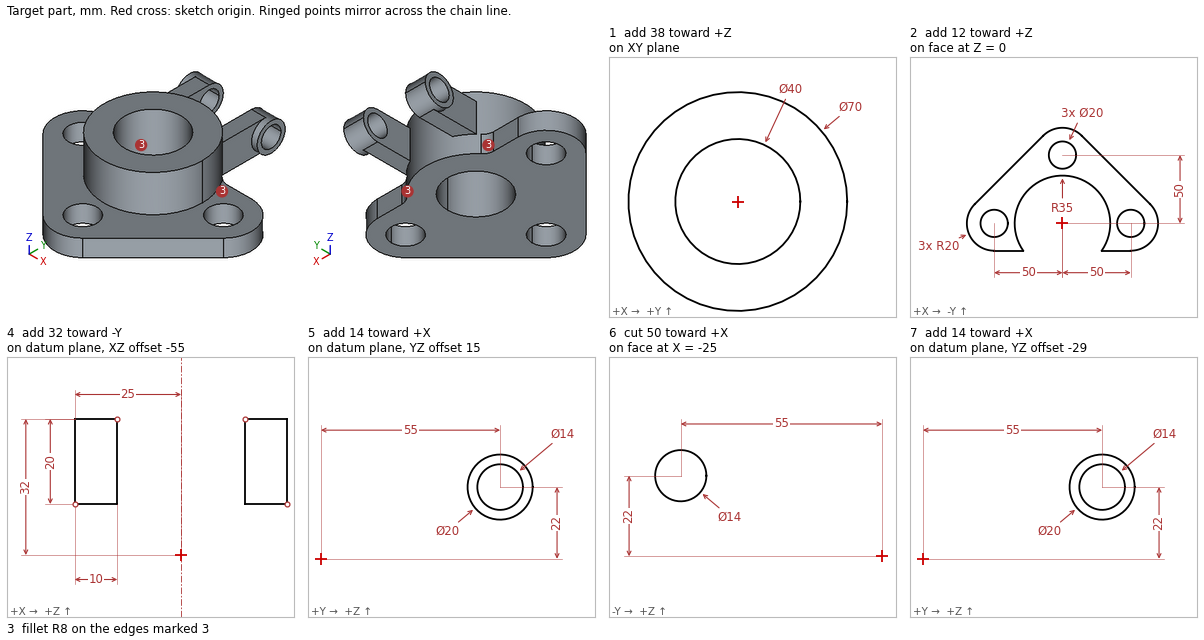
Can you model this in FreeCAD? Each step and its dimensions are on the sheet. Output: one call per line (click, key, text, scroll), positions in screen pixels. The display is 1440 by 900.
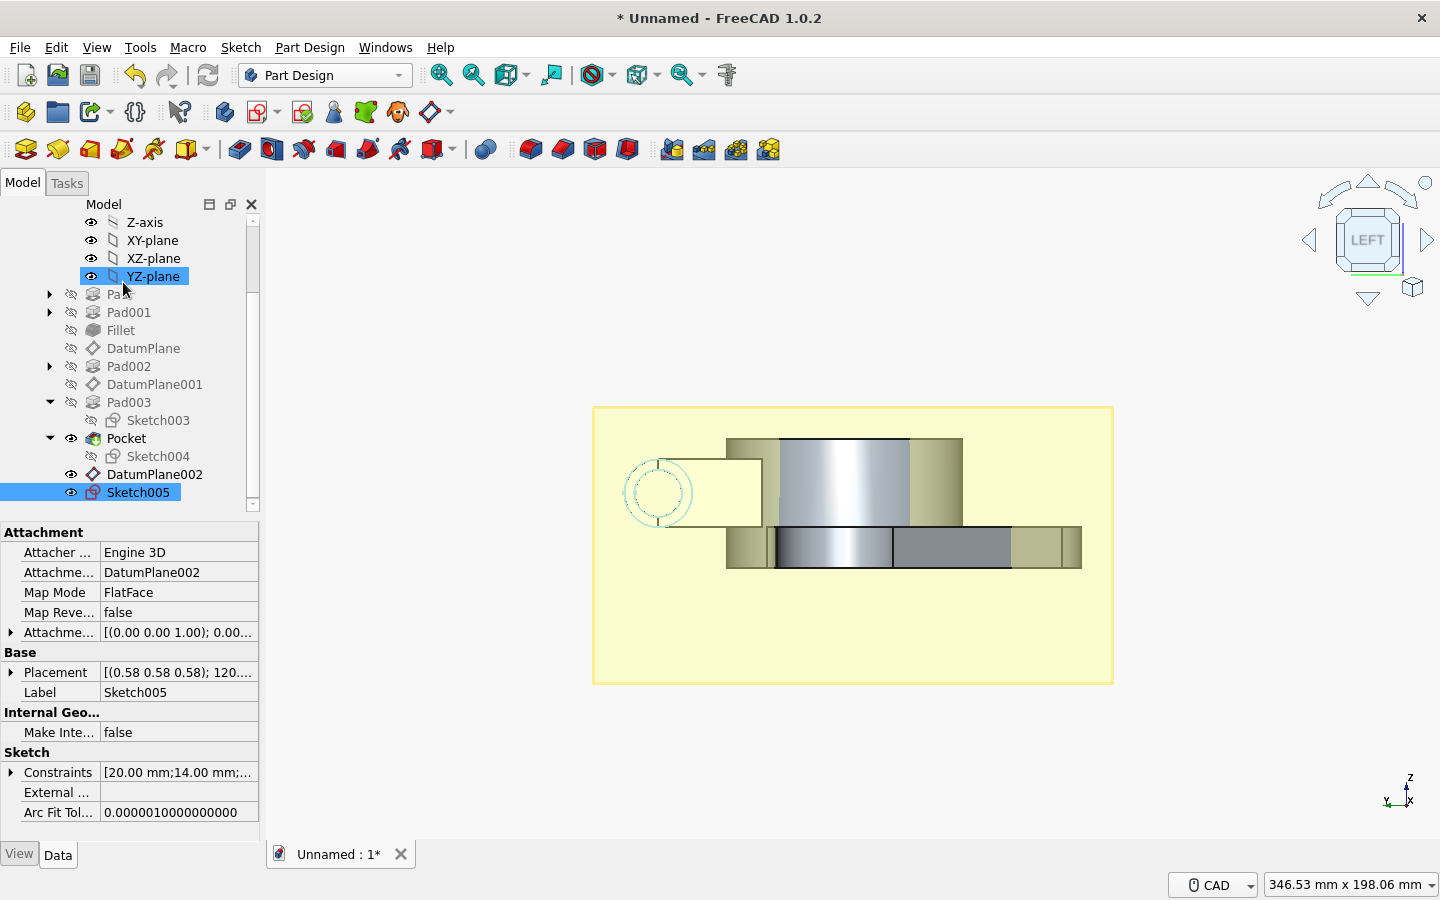
click(26, 150)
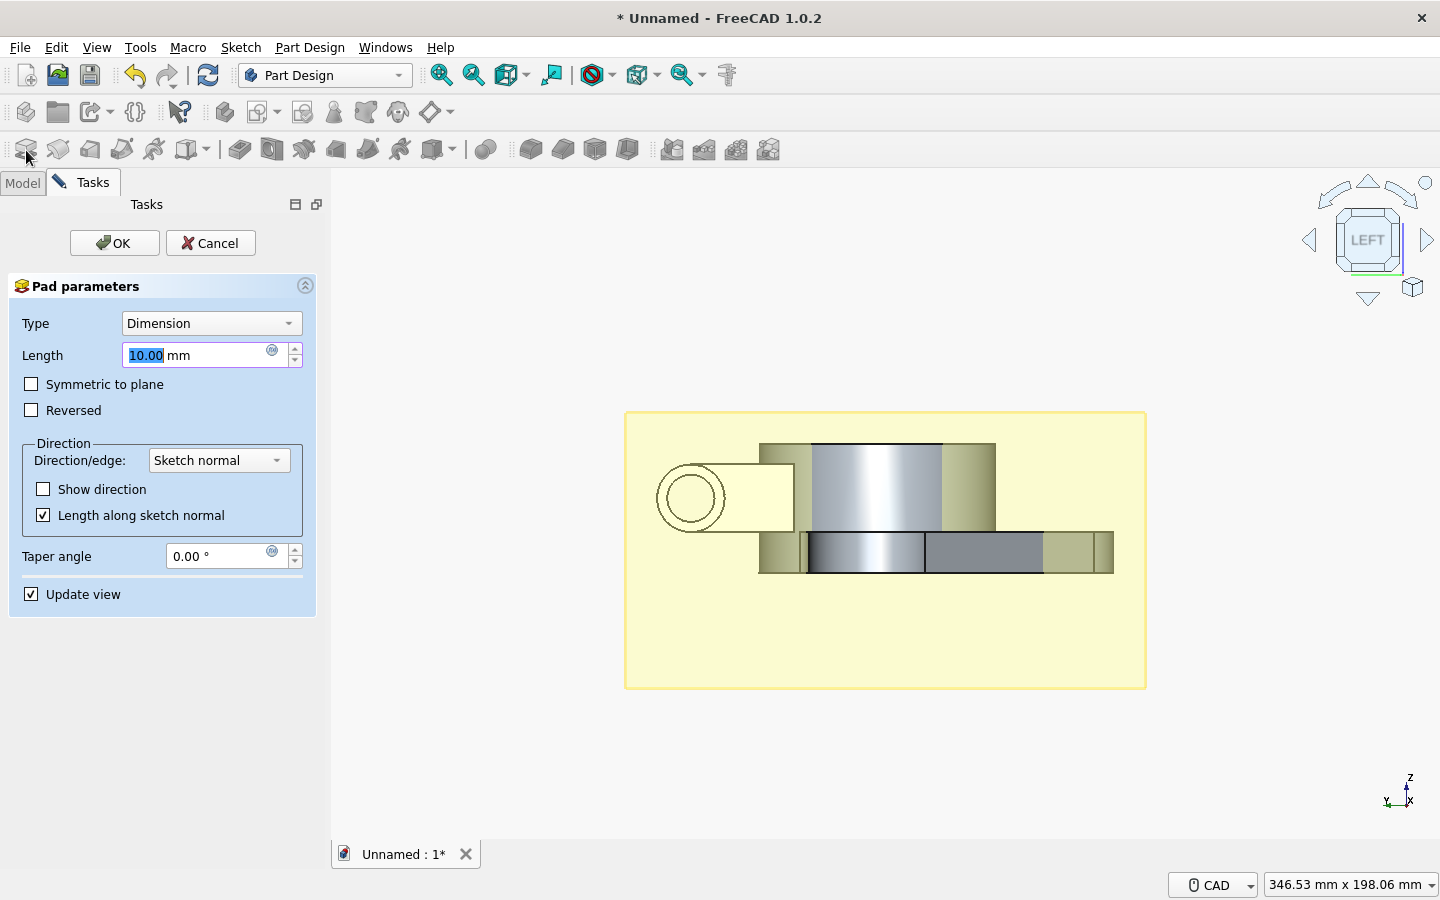
text(14)
key(Tab)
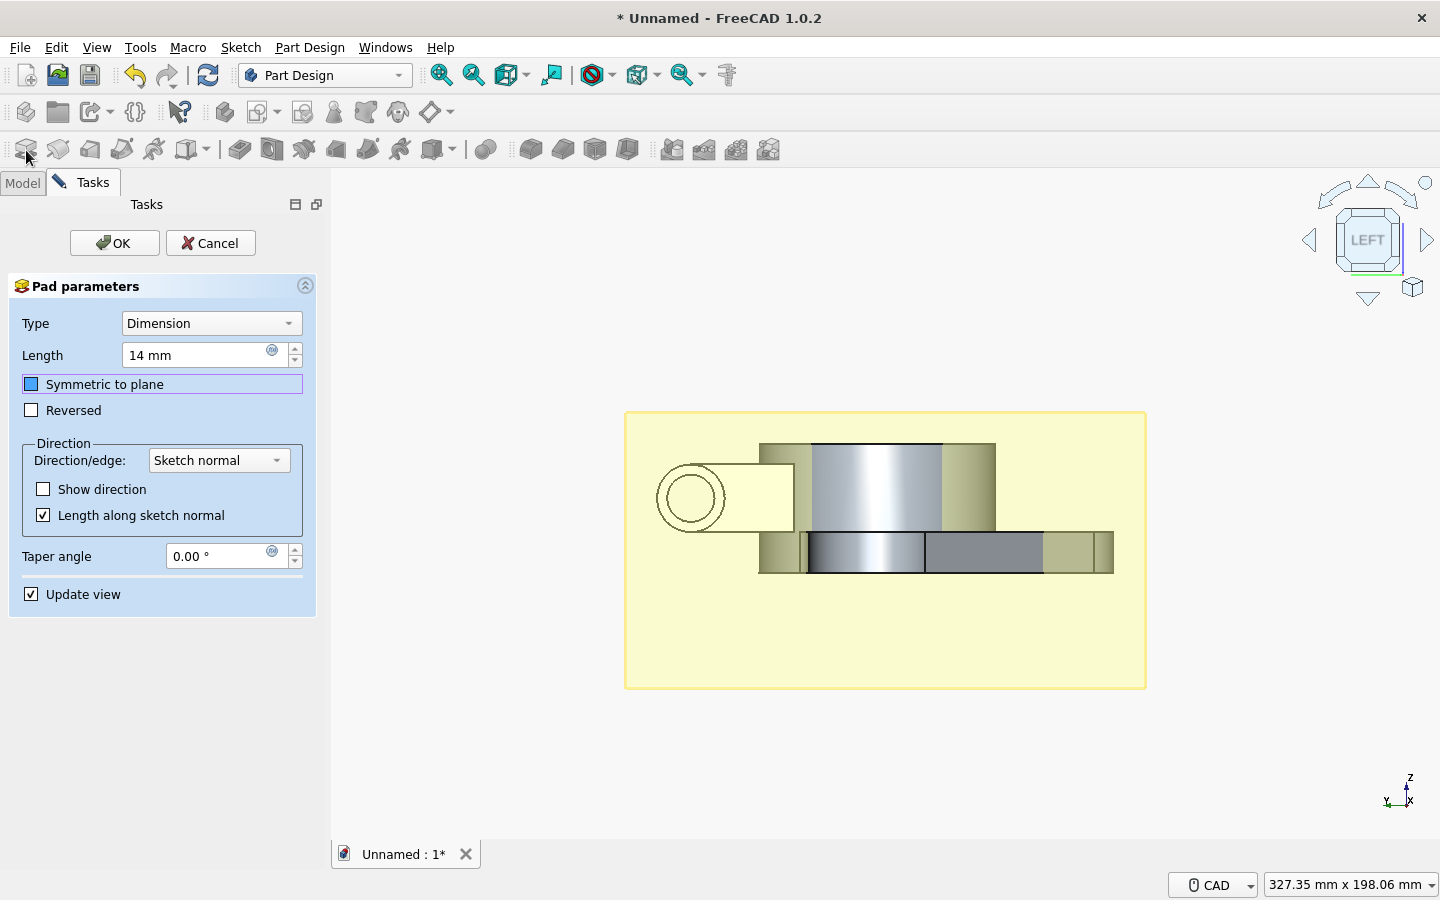
click(115, 243)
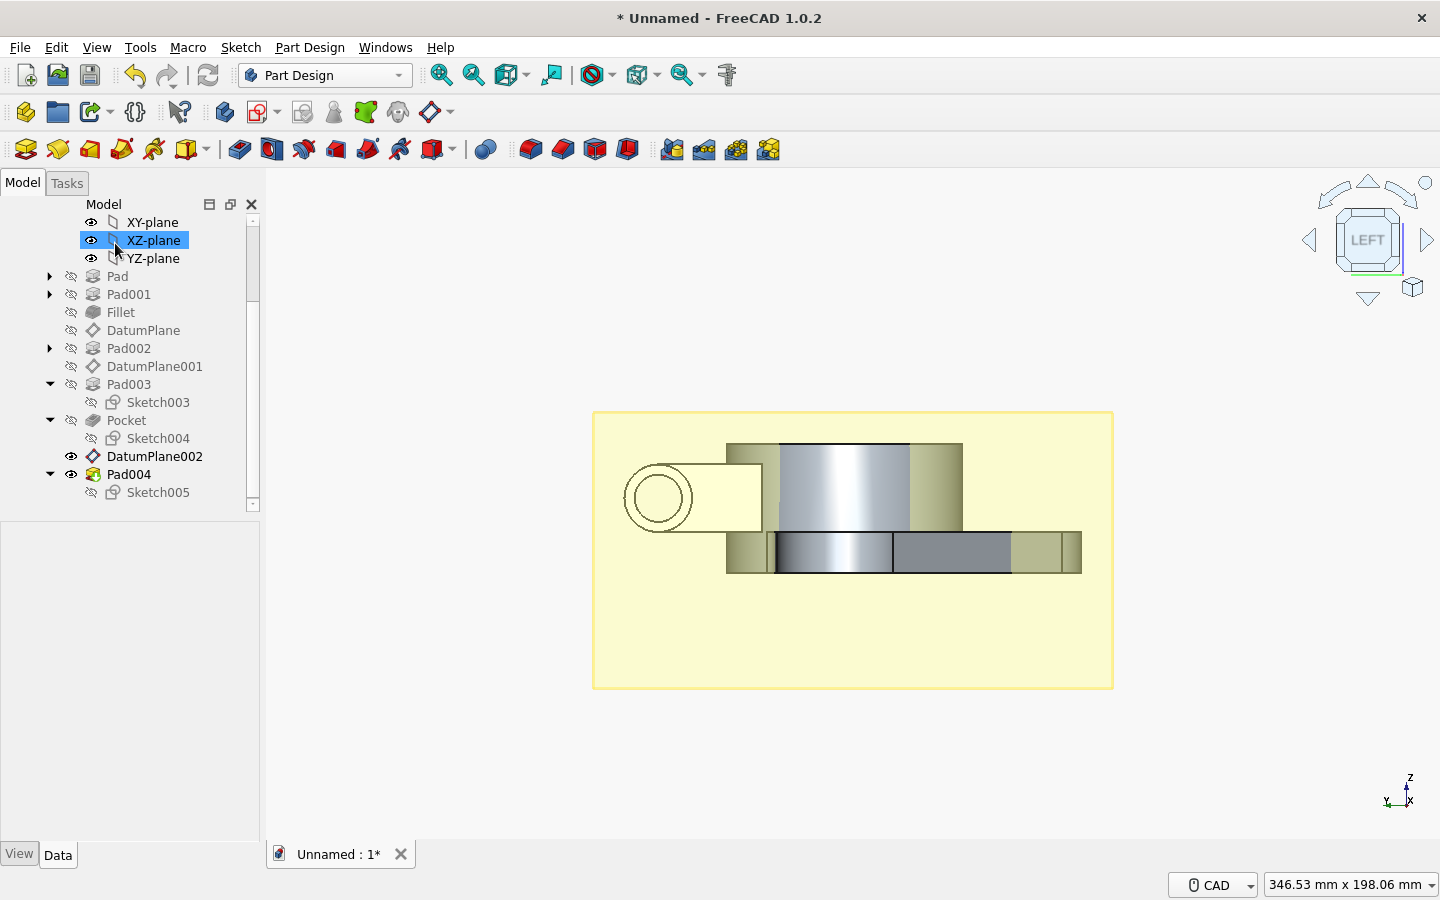
click(116, 456)
key(space)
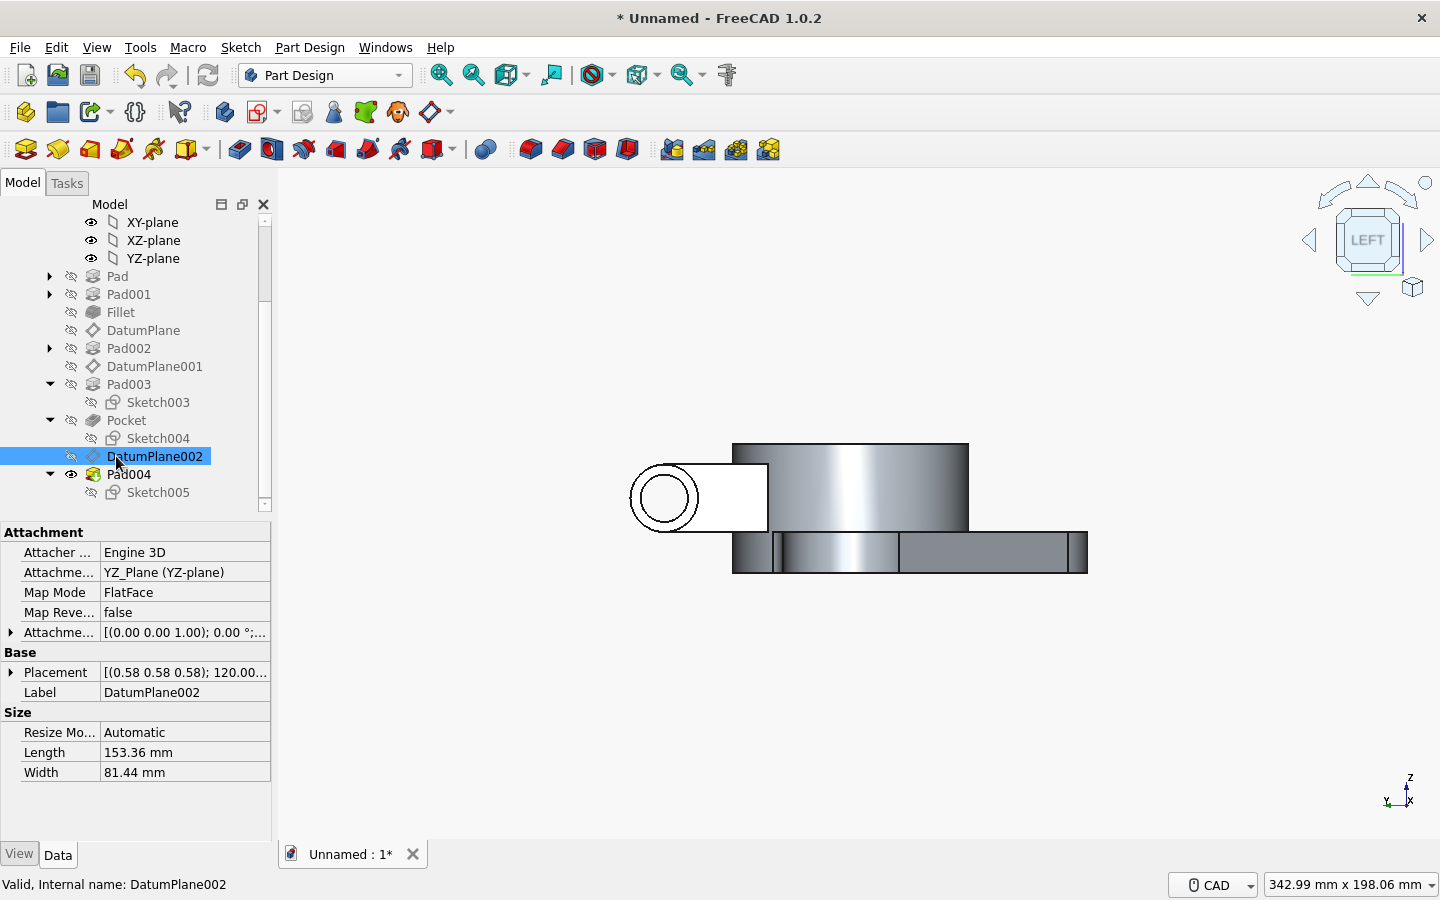
key(0)